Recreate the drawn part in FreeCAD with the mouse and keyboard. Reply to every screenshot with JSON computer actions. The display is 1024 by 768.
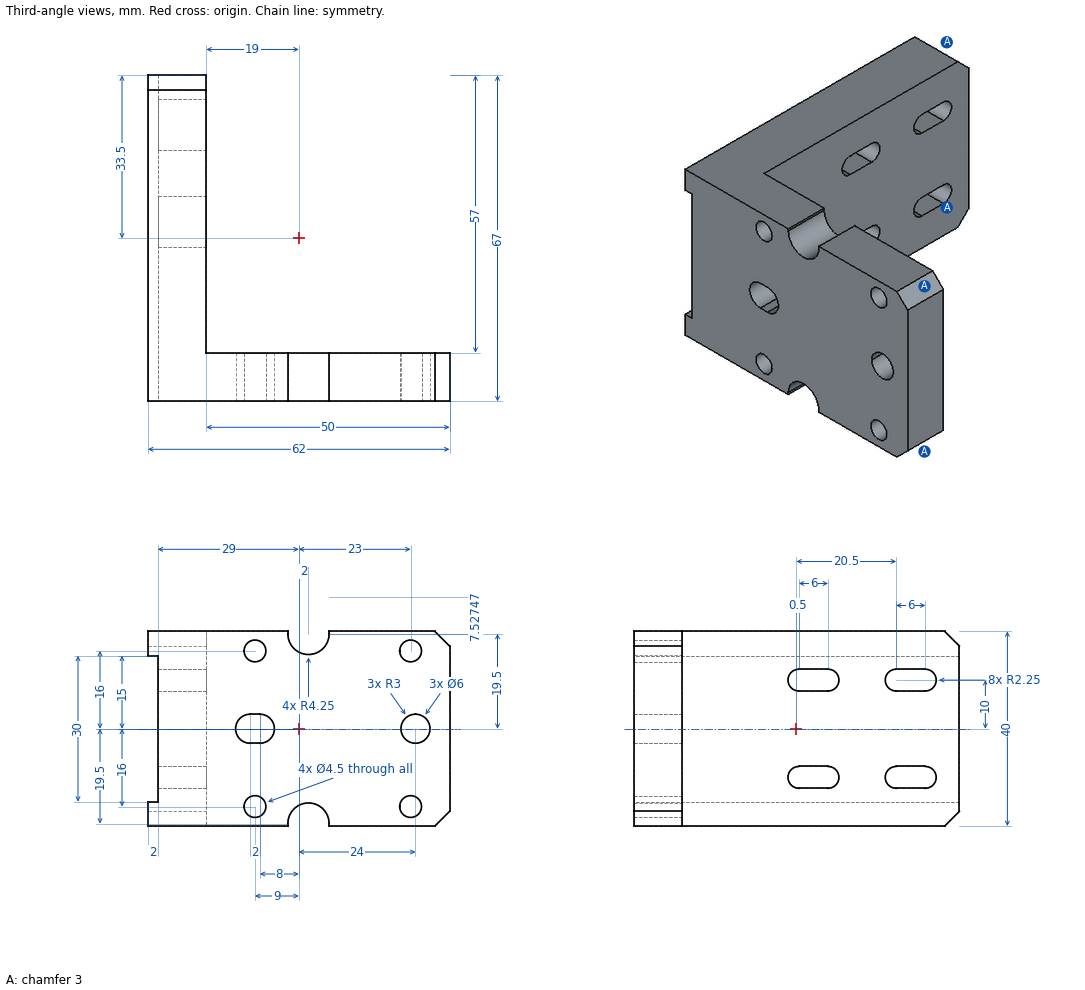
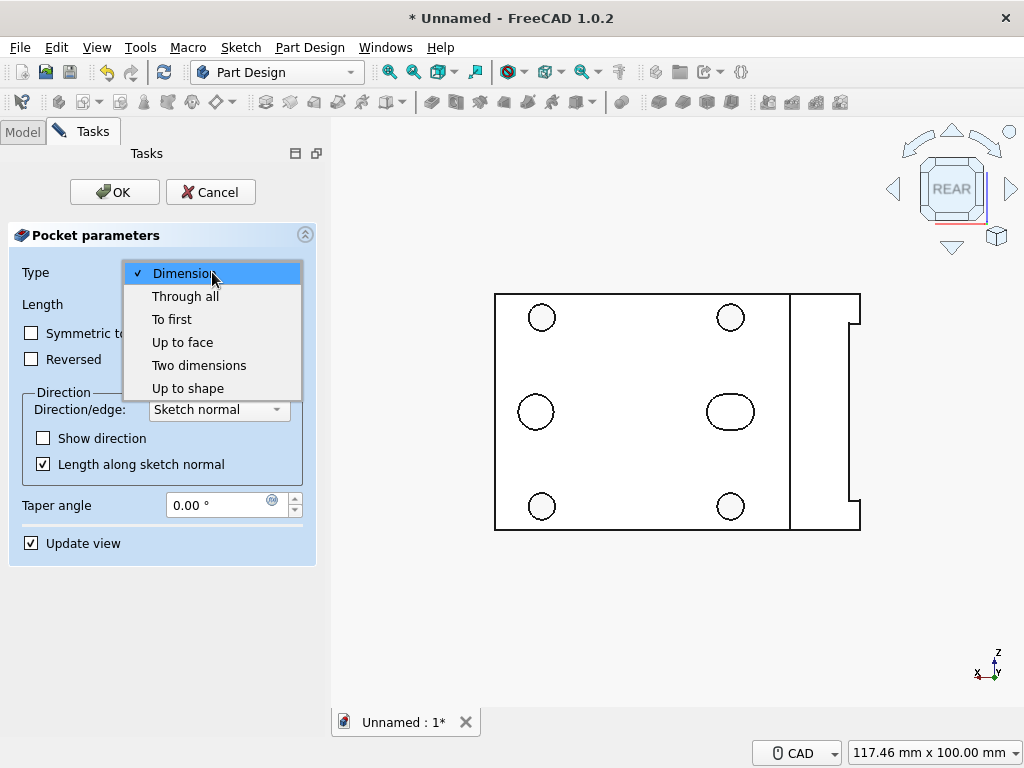
{"action": "left_click", "coordinate": [212, 296]}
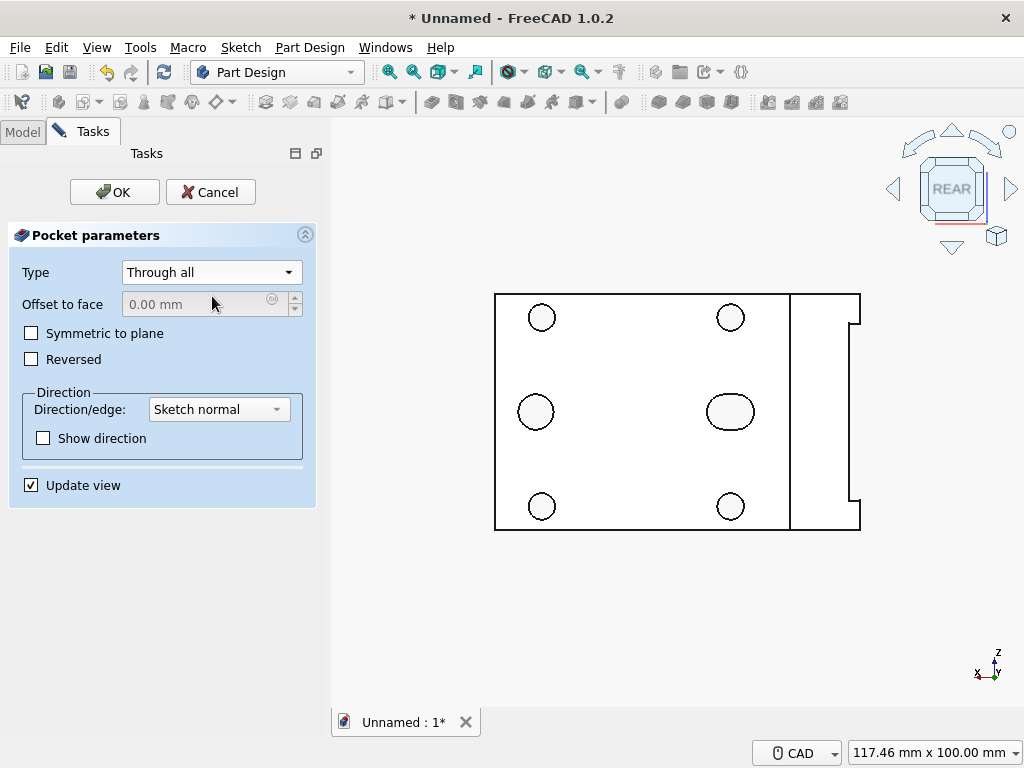
{"action": "left_click", "coordinate": [115, 192]}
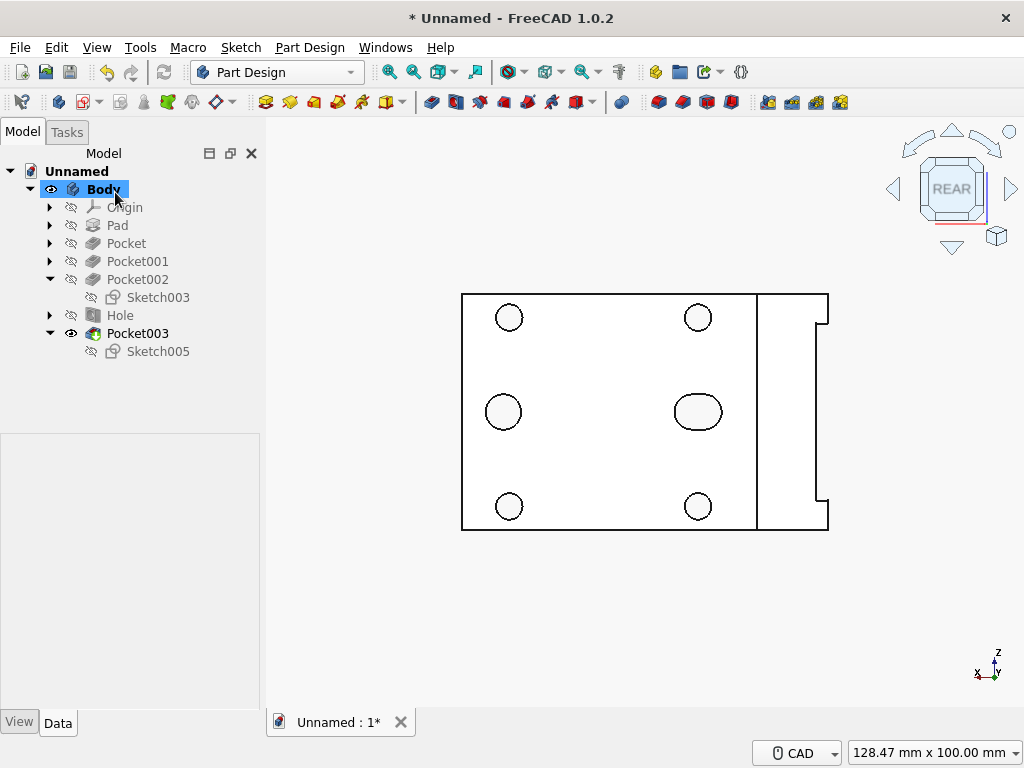
{"action": "left_click", "coordinate": [793, 529]}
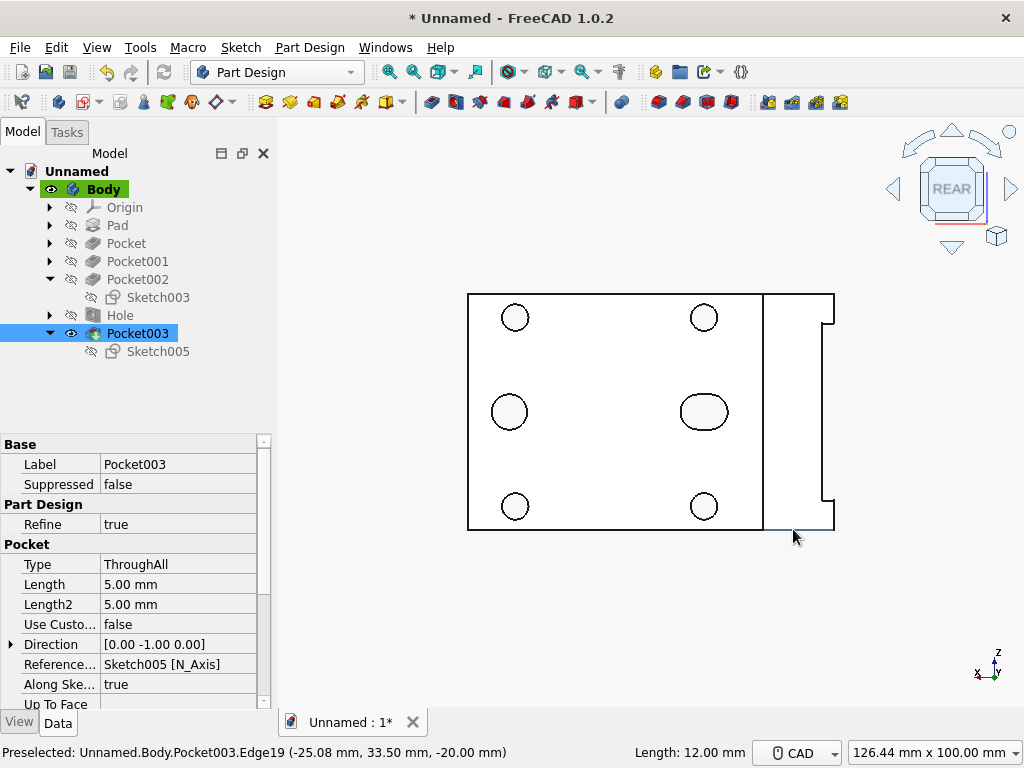
{"action": "left_click", "coordinate": [799, 293], "text": "ctrl"}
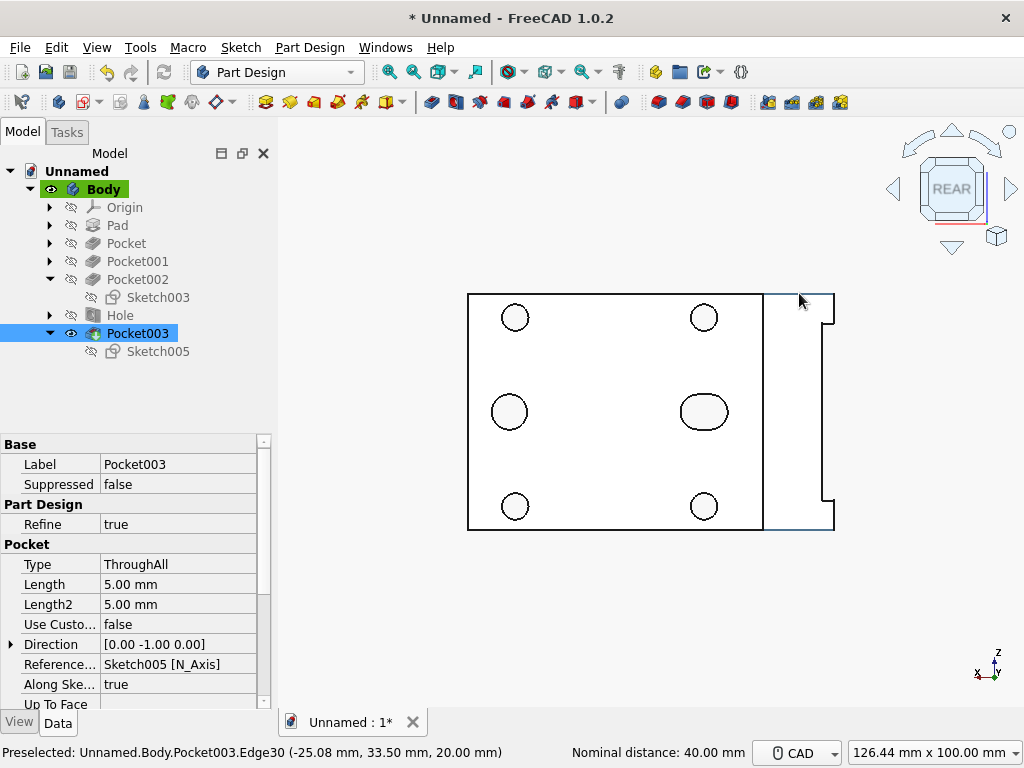
{"action": "key", "text": "0"}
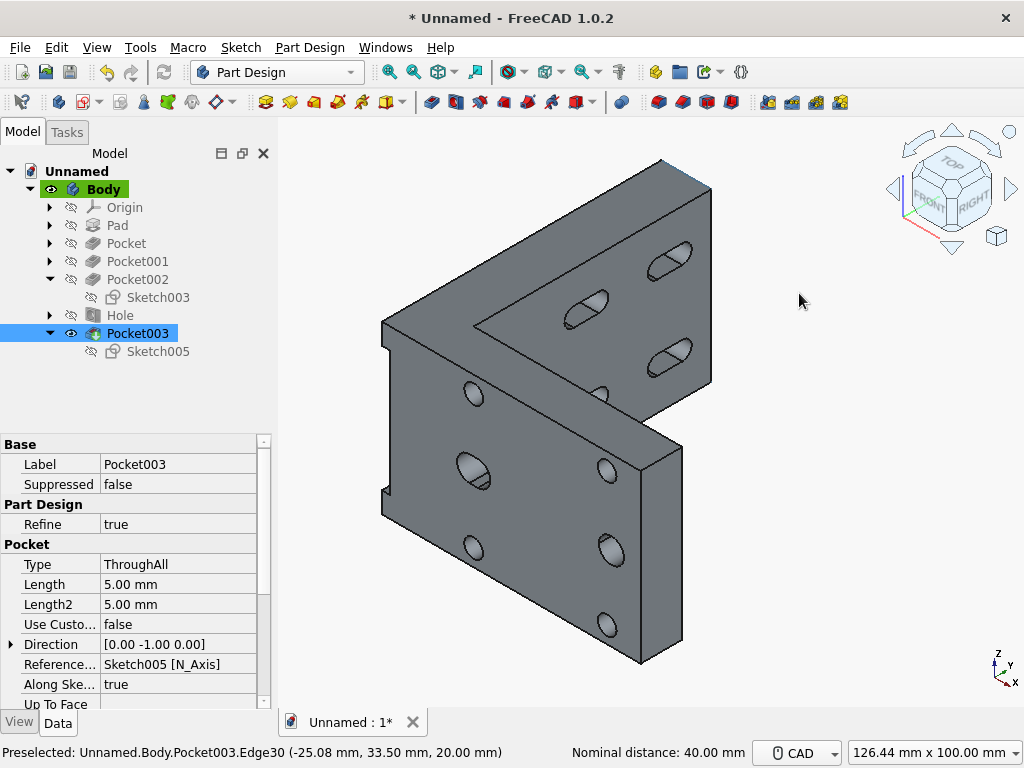
{"action": "left_click", "coordinate": [661, 458], "text": "ctrl"}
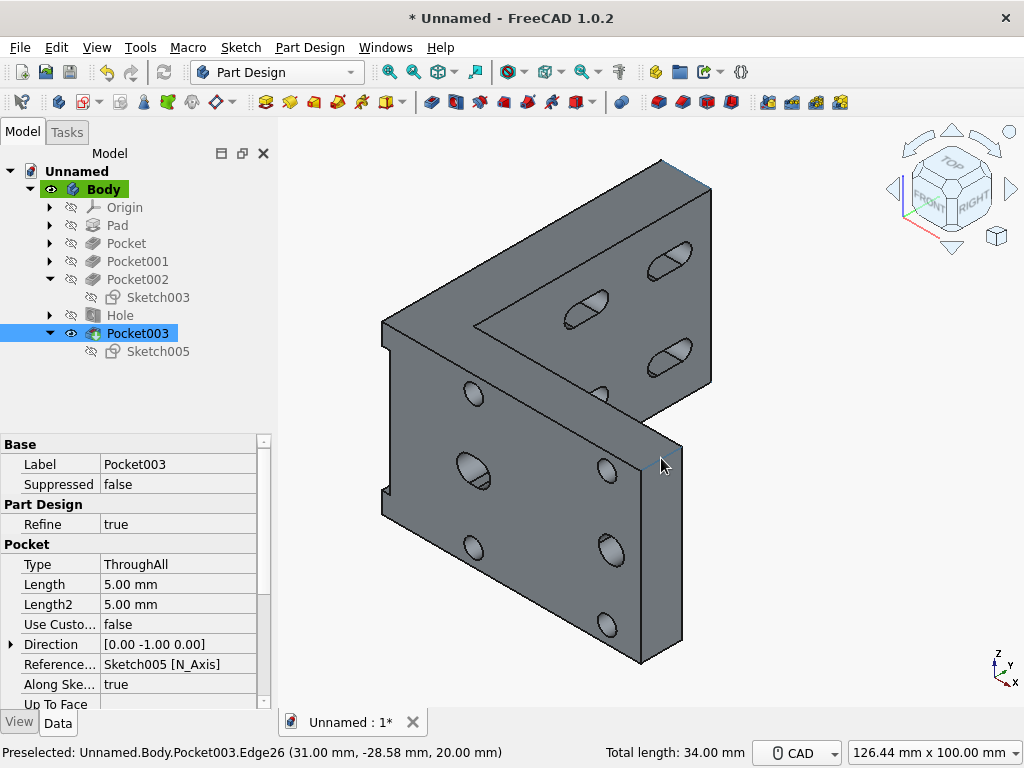
{"action": "key", "text": "2"}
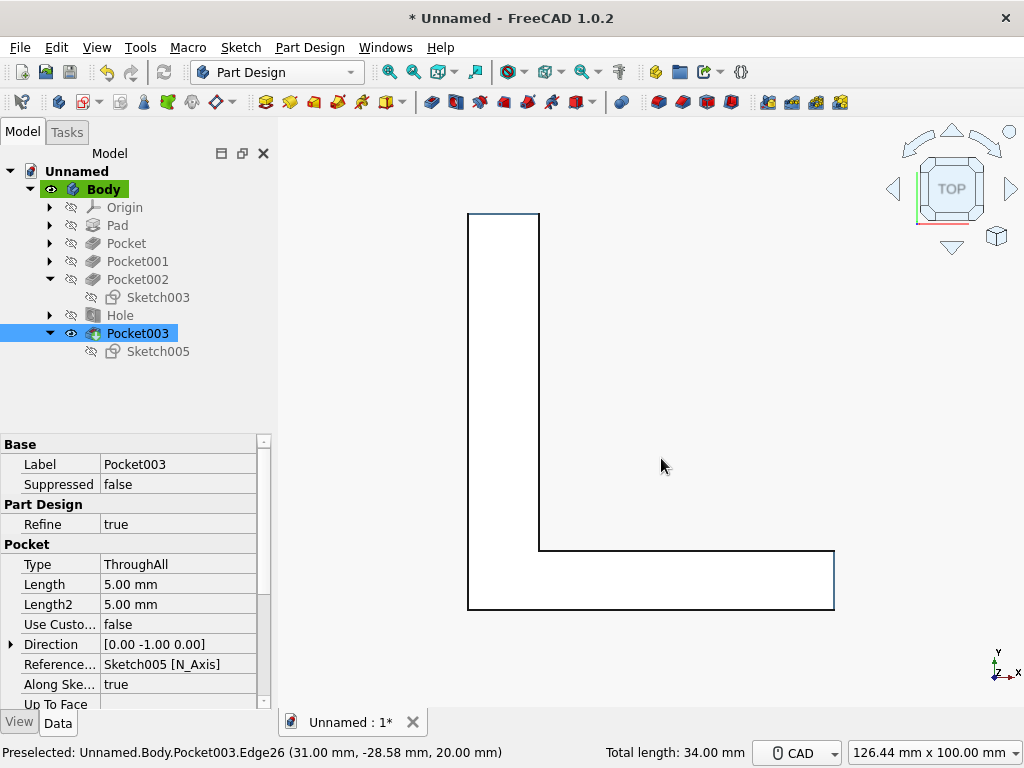
{"action": "key", "text": "1"}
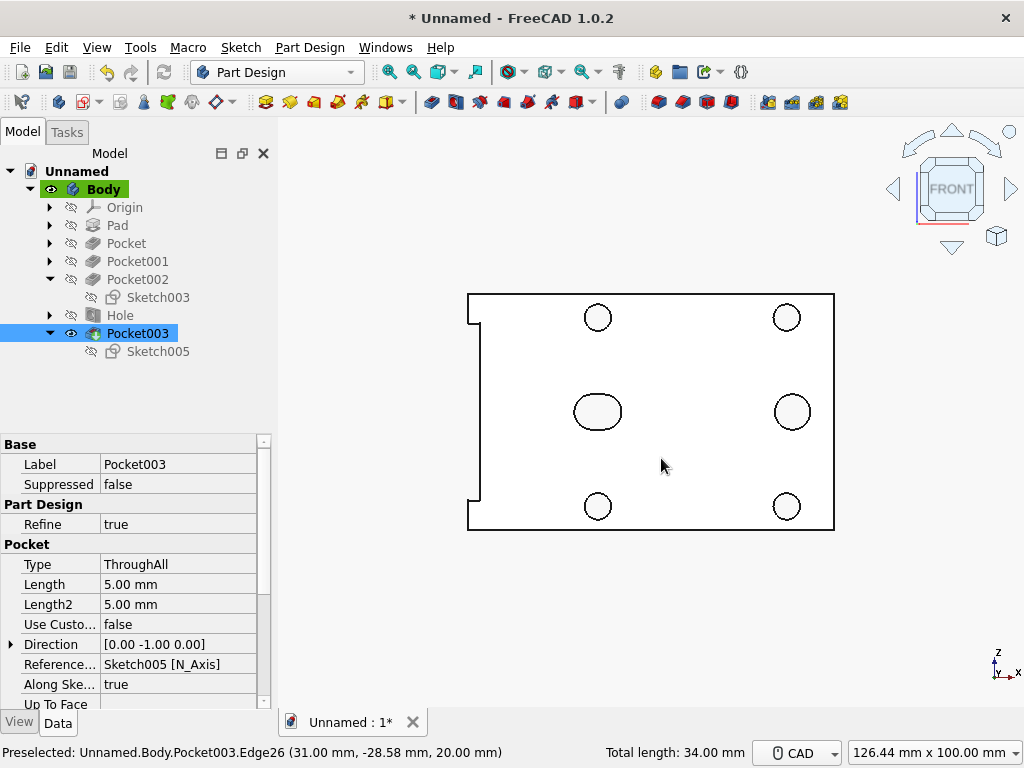
{"action": "key", "text": "3"}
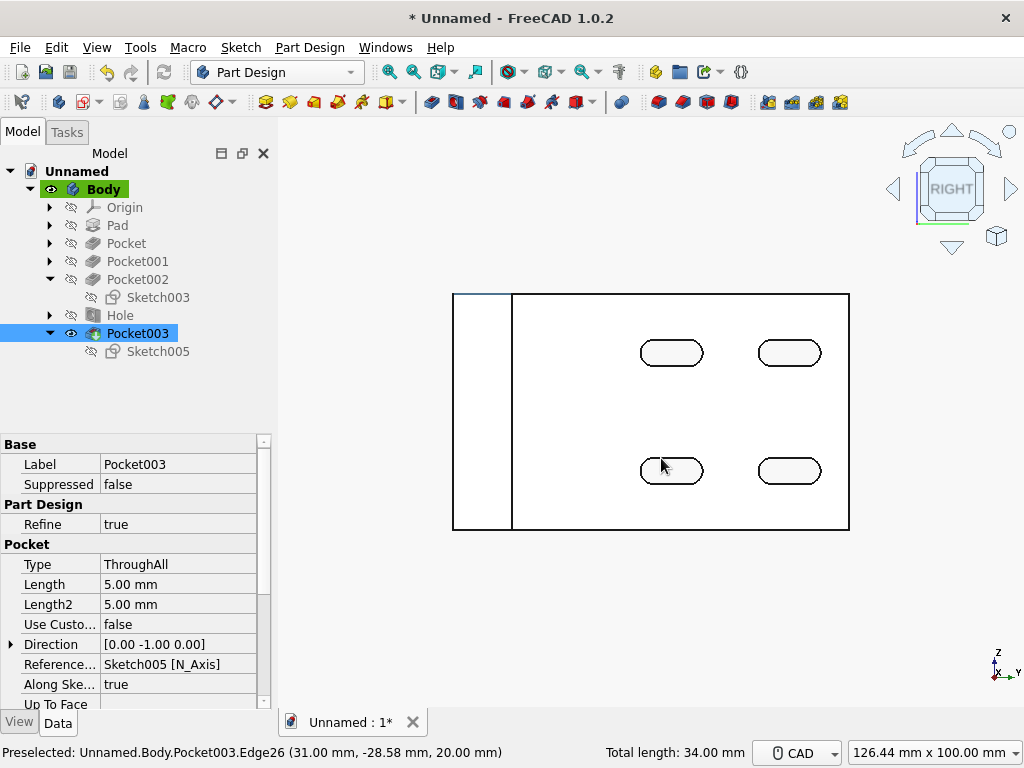
{"action": "left_click", "coordinate": [483, 529], "text": "ctrl"}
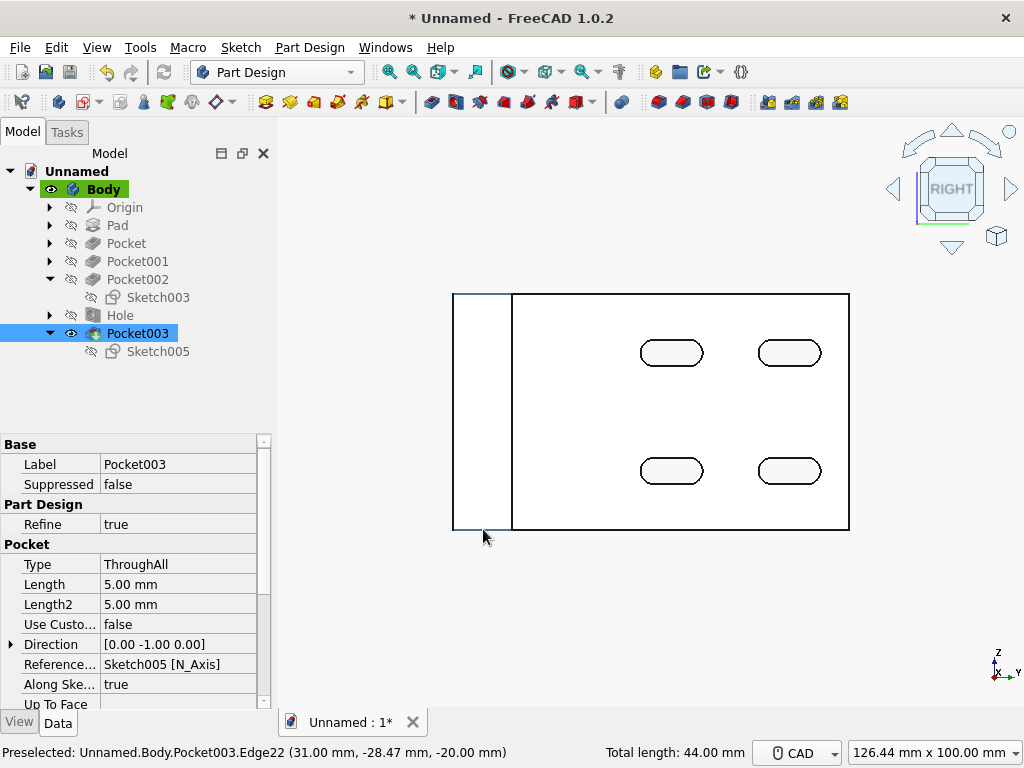
{"action": "left_click", "coordinate": [684, 102]}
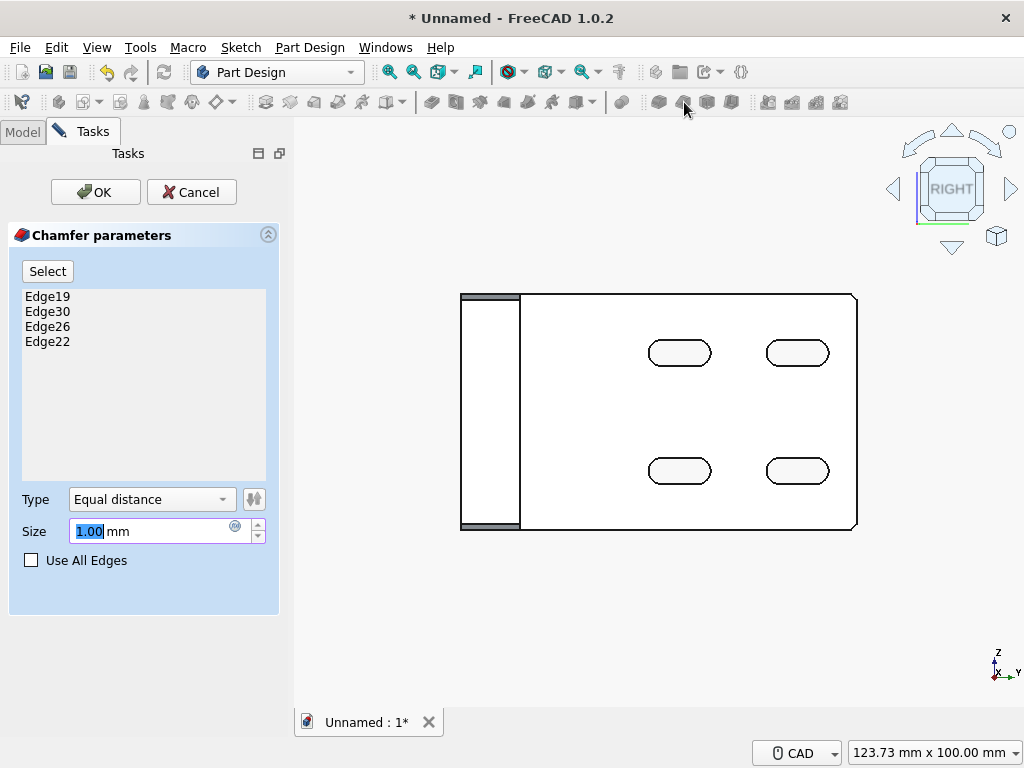
{"action": "type", "text": "3"}
{"action": "key", "text": "Tab"}